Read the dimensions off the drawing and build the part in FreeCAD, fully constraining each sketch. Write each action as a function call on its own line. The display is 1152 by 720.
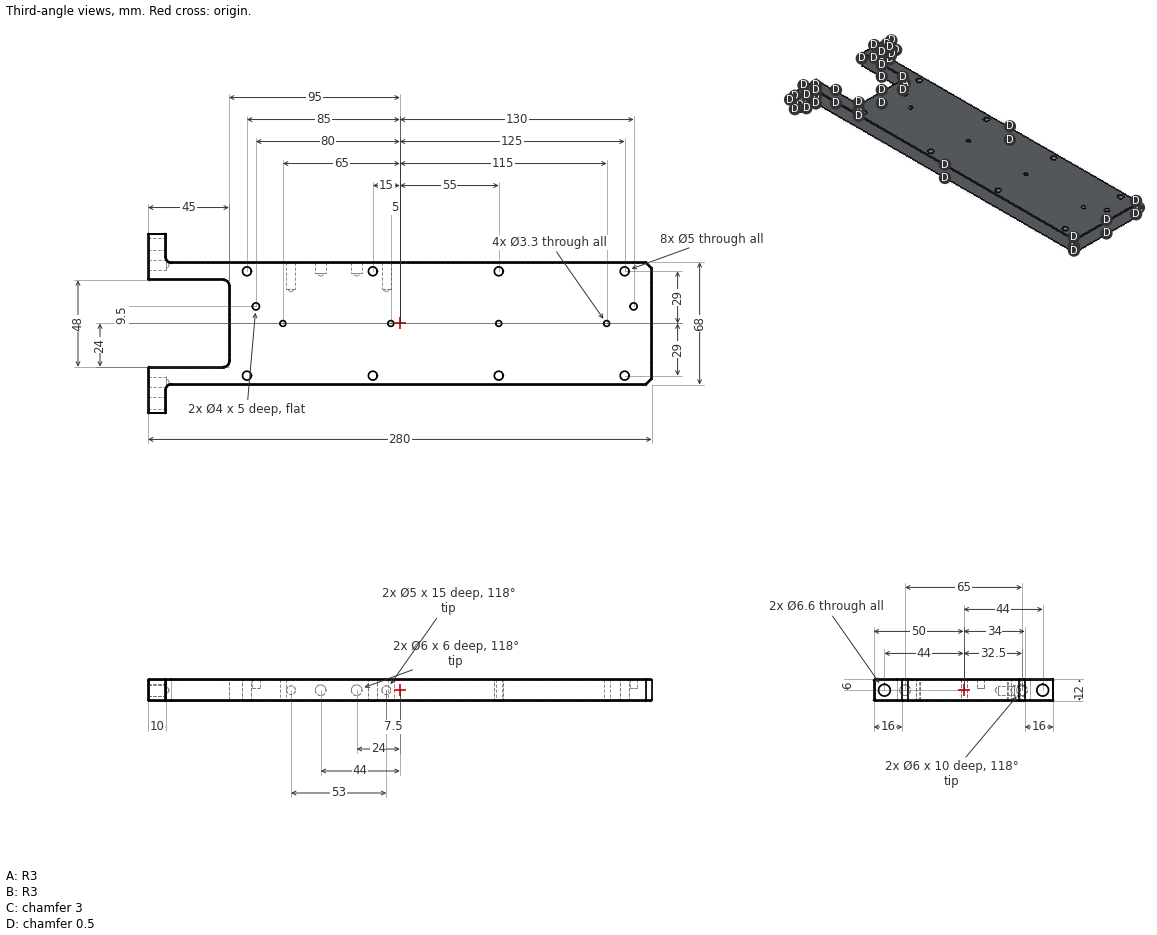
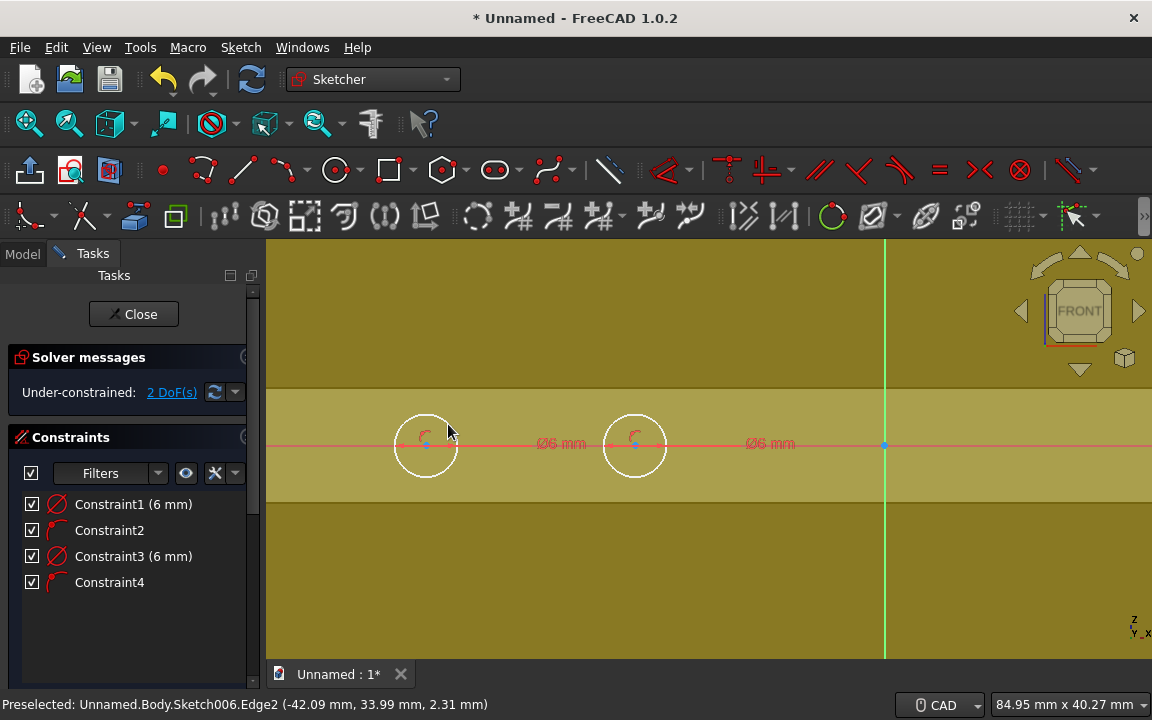
click(664, 170)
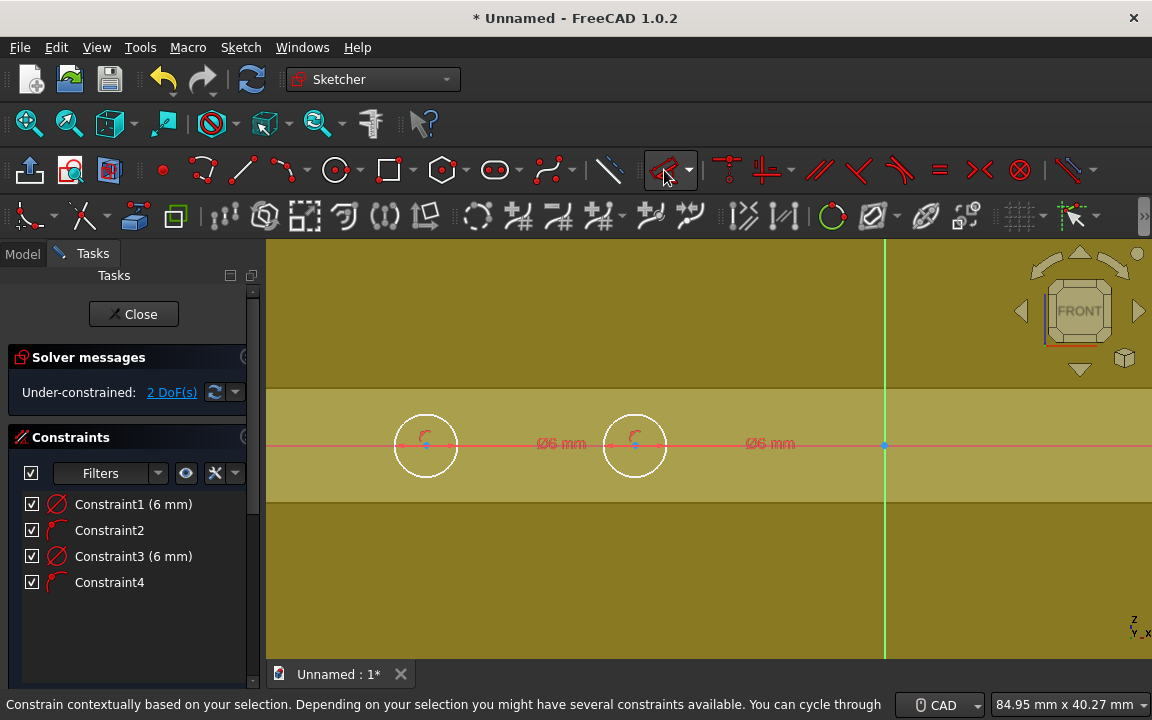
click(635, 446)
click(760, 480)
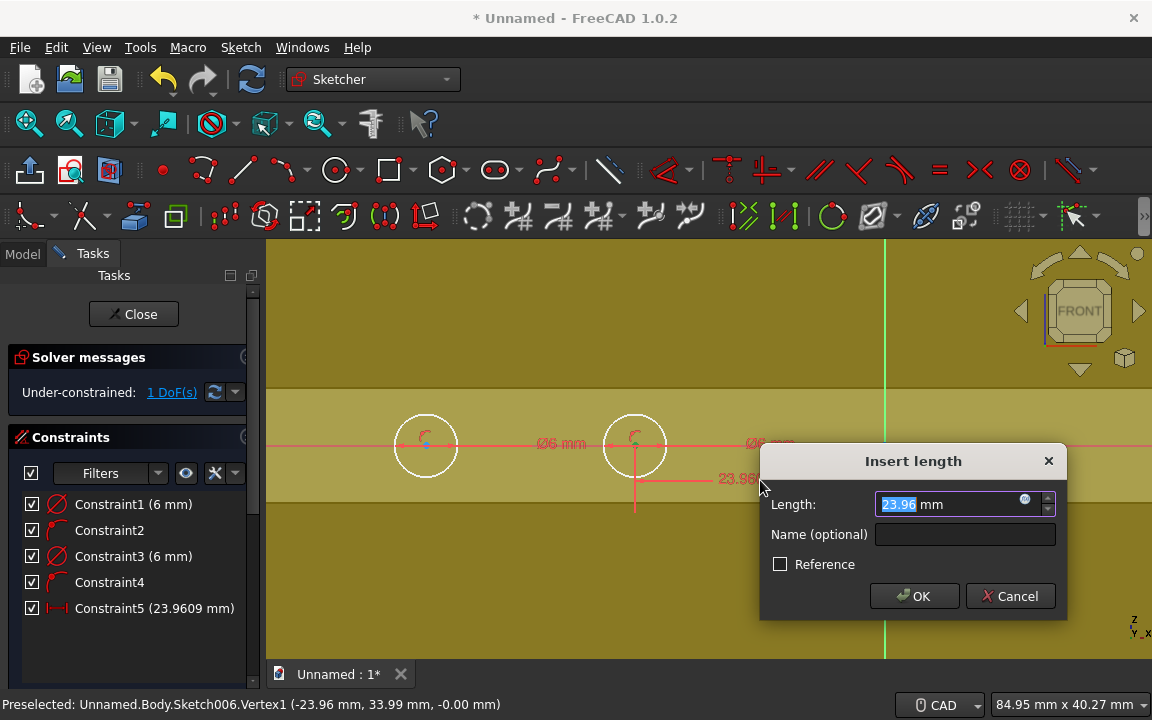
text(24)
key(Return)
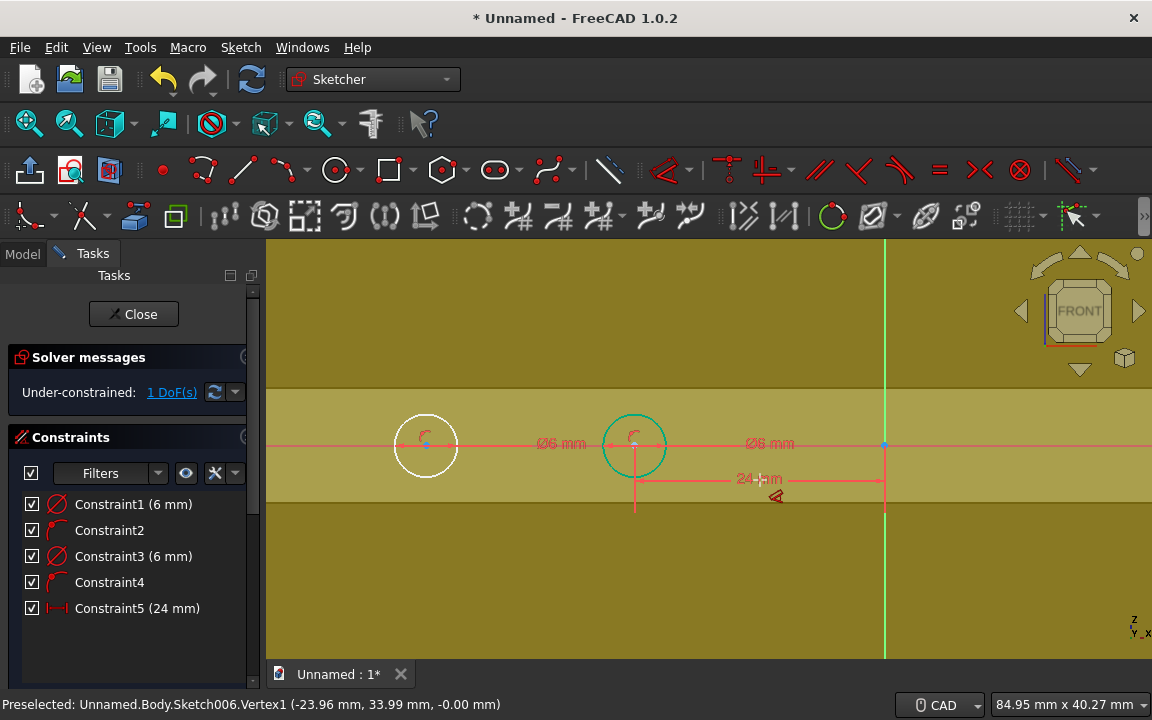
click(426, 446)
click(550, 480)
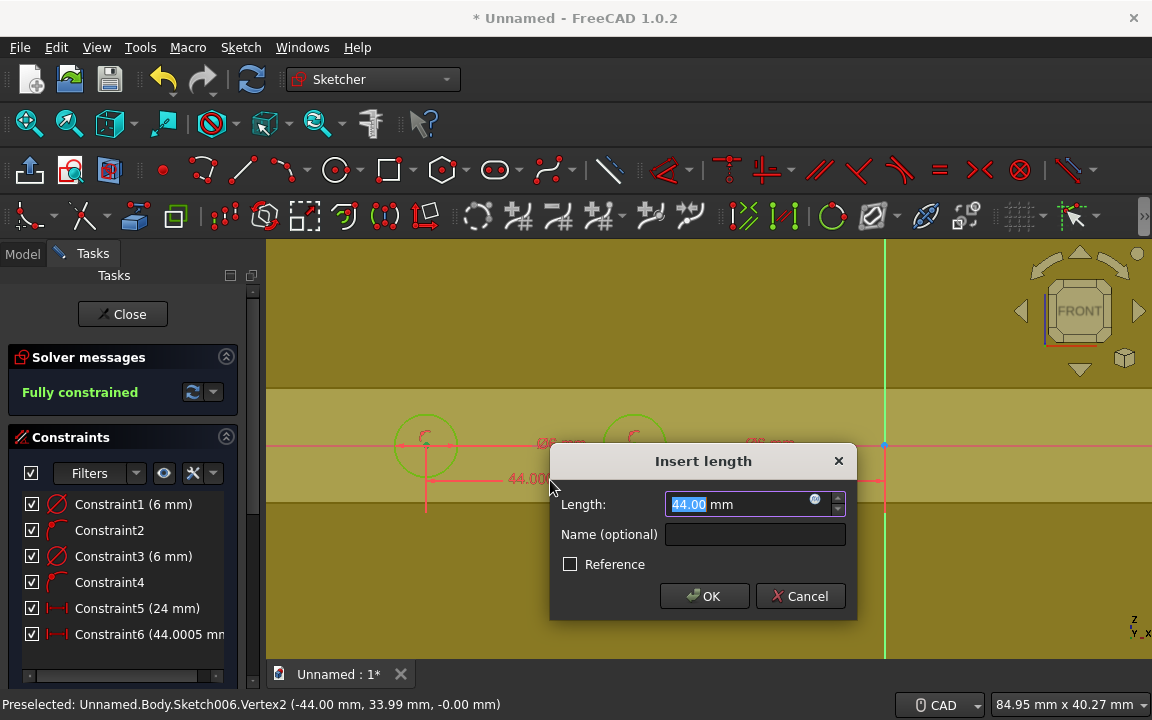
text(44)
key(Return)
key(Escape)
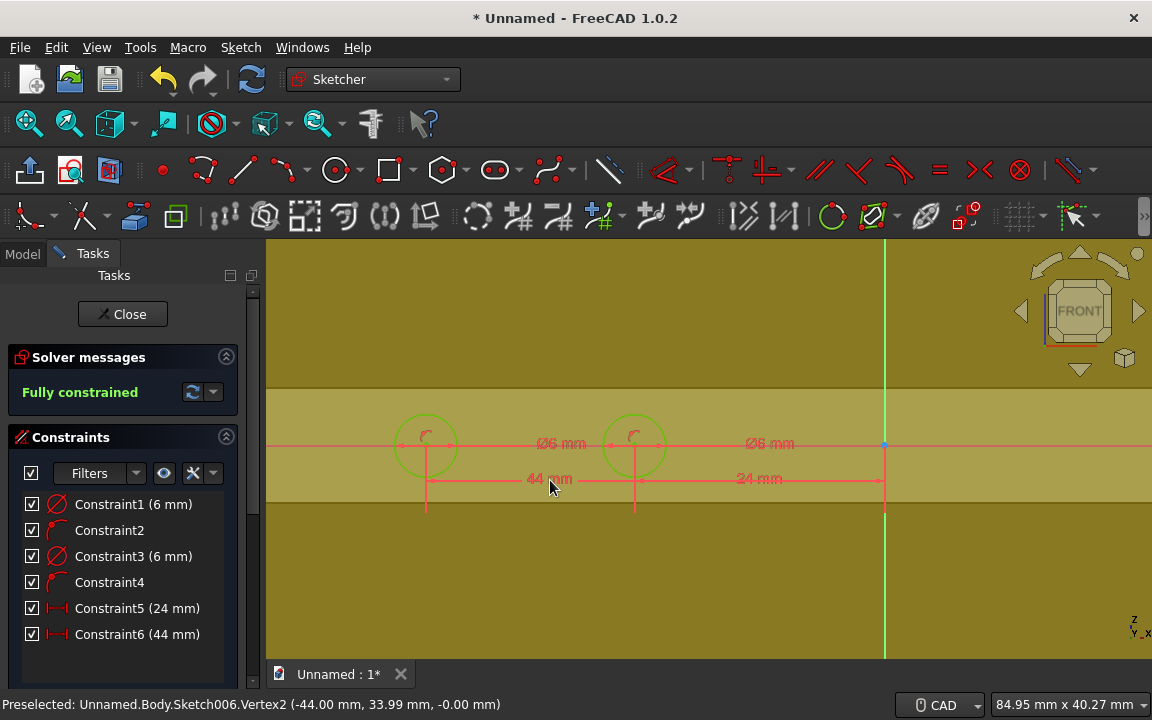
click(123, 314)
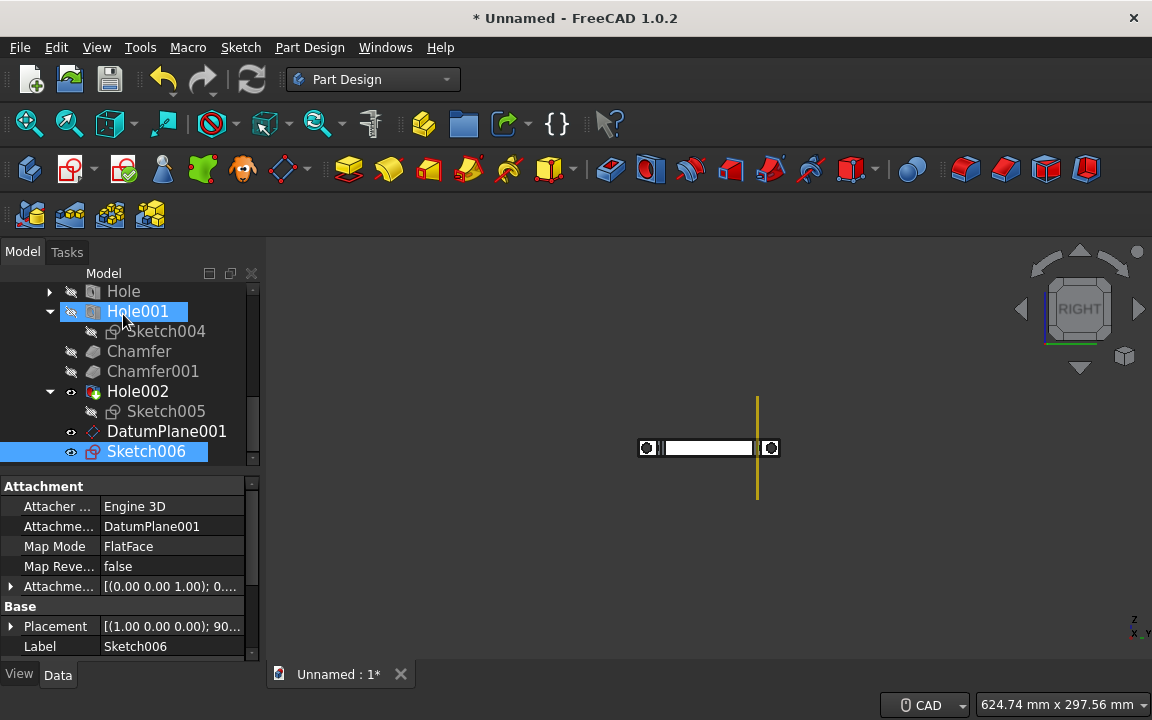
click(652, 170)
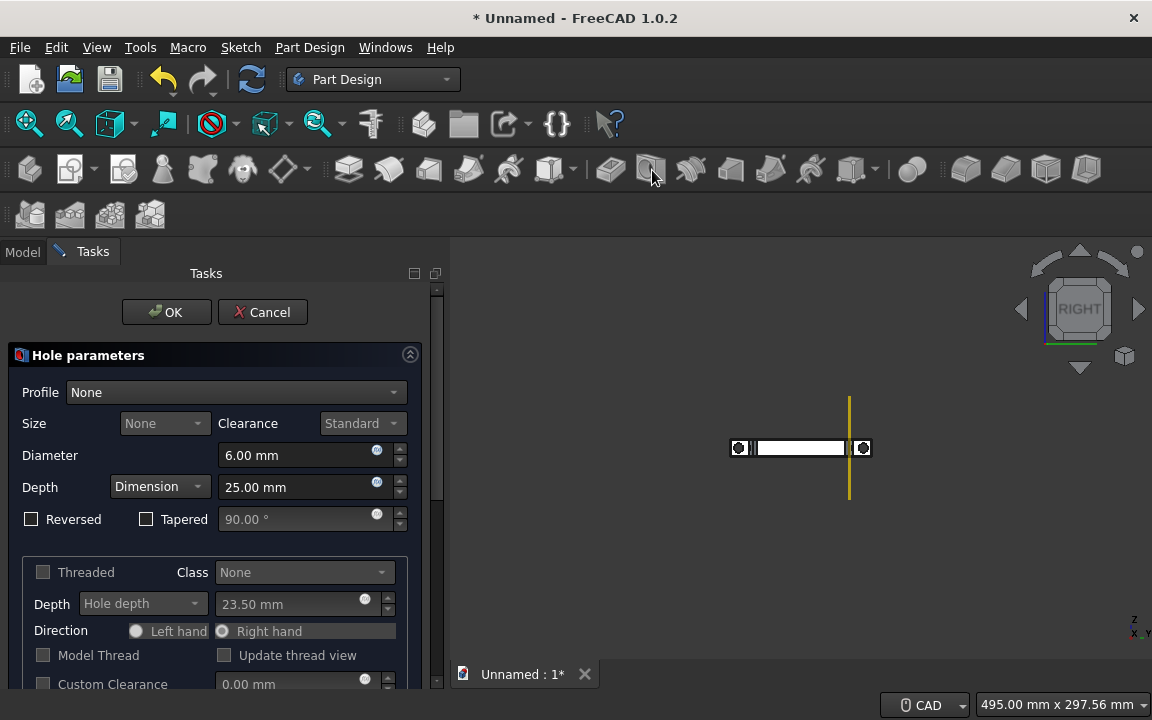
triple_click(305, 455)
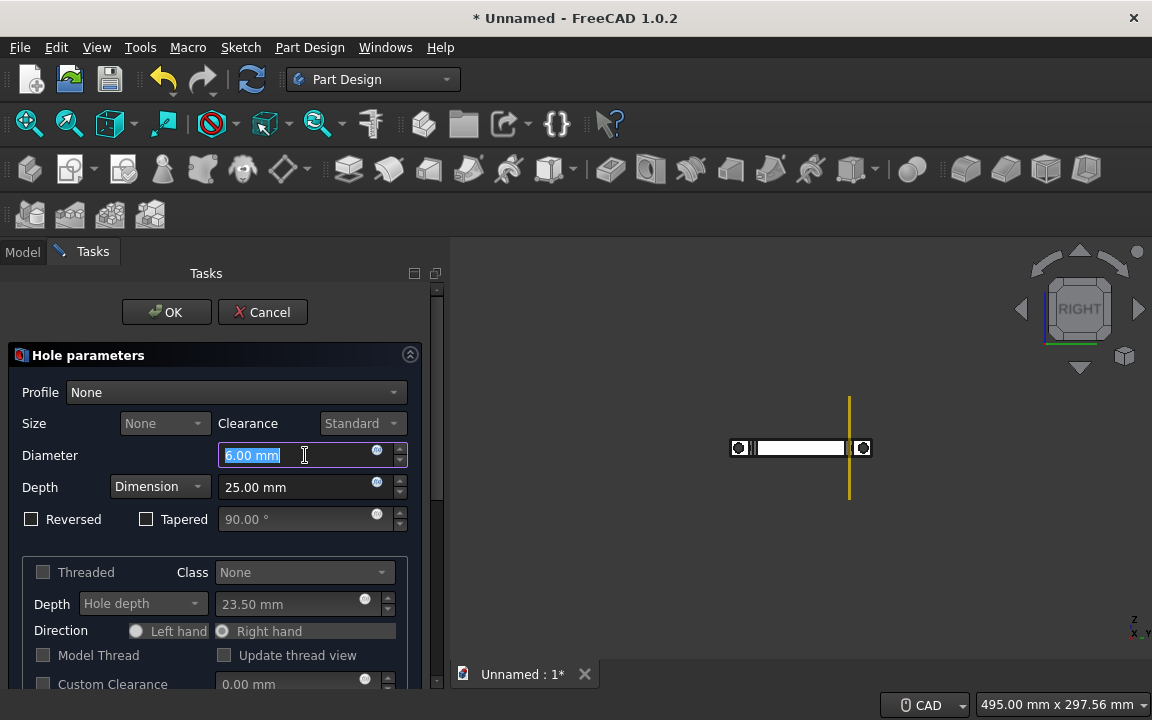
text(6)
key(Tab)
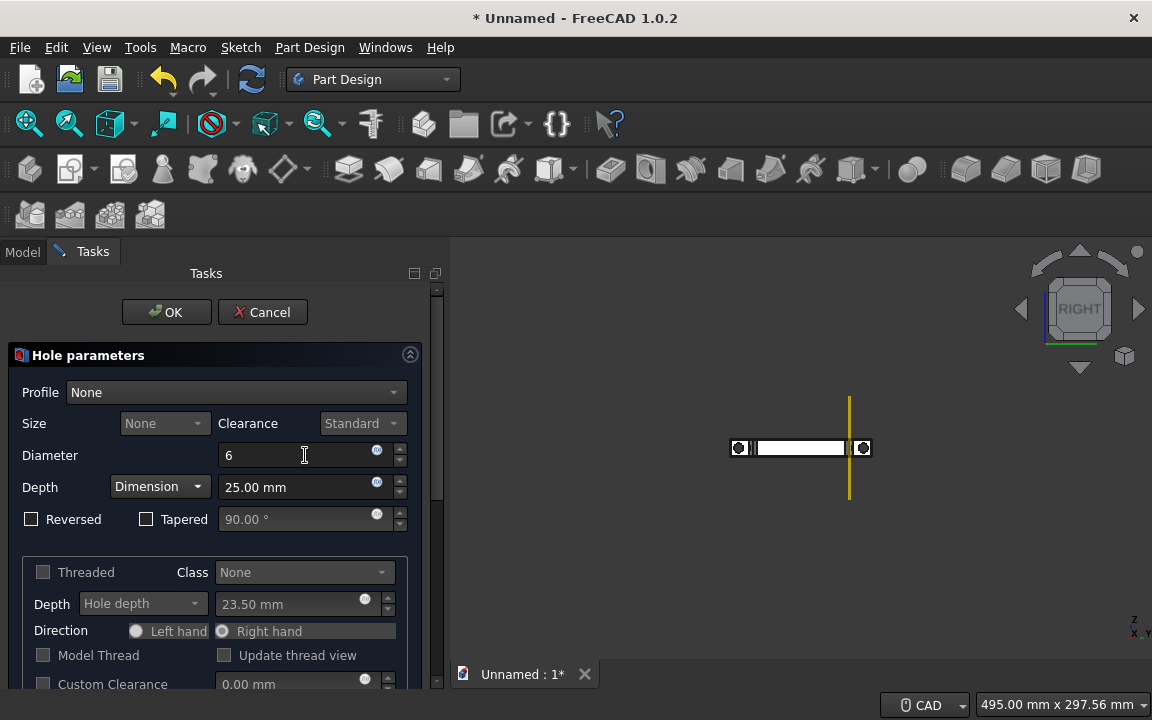
triple_click(305, 487)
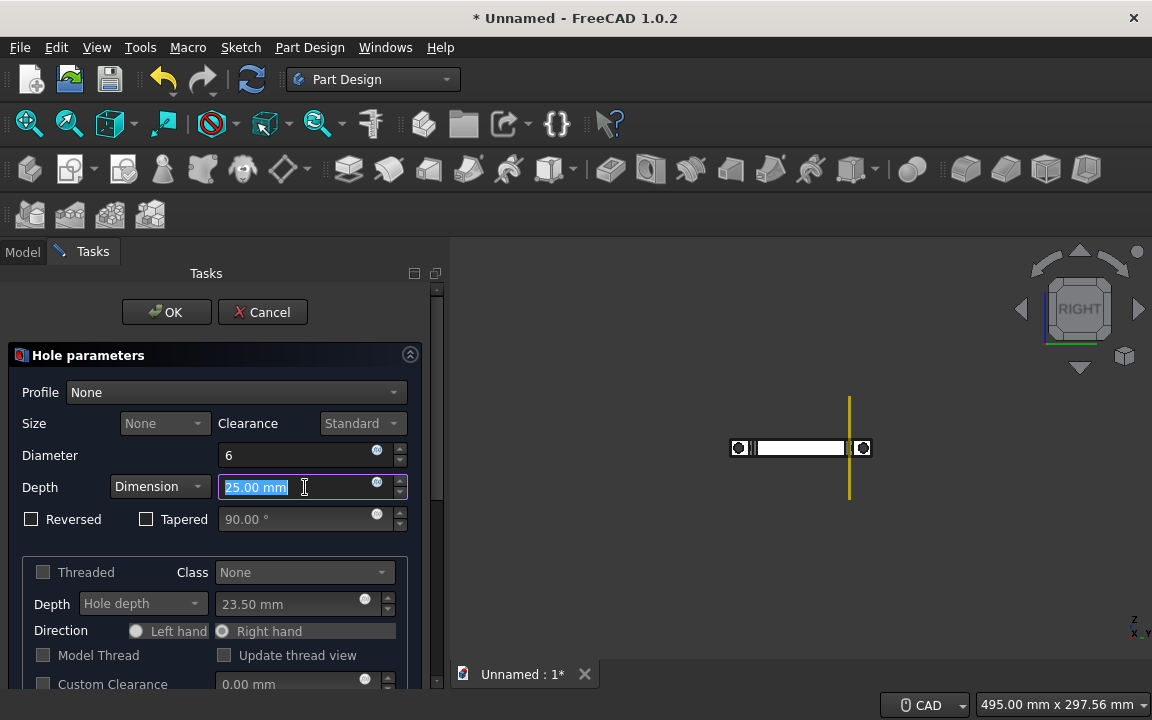
text(6)
key(Tab)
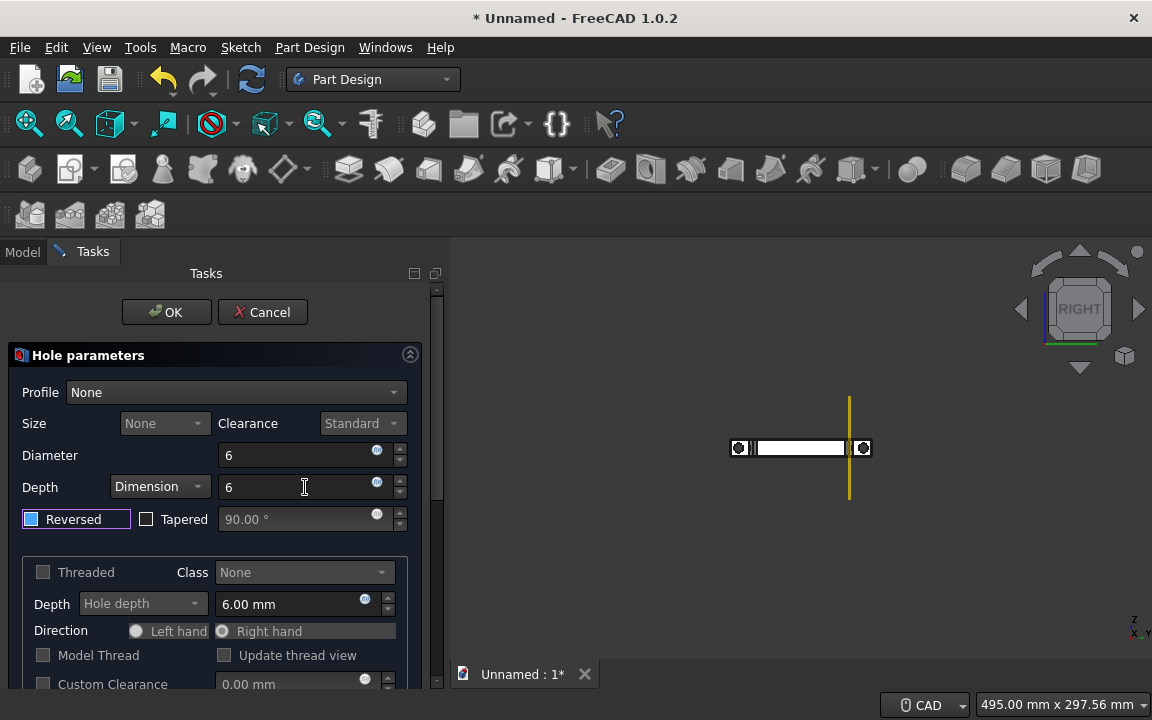
click(30, 519)